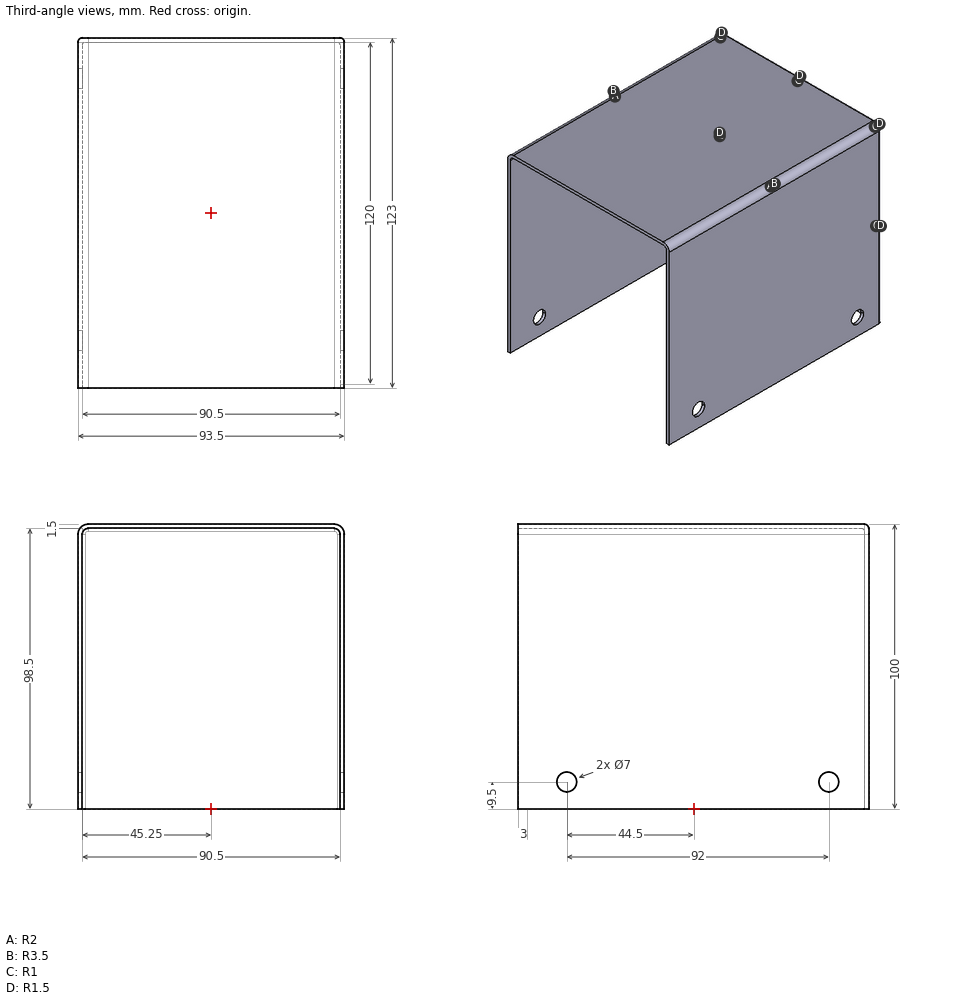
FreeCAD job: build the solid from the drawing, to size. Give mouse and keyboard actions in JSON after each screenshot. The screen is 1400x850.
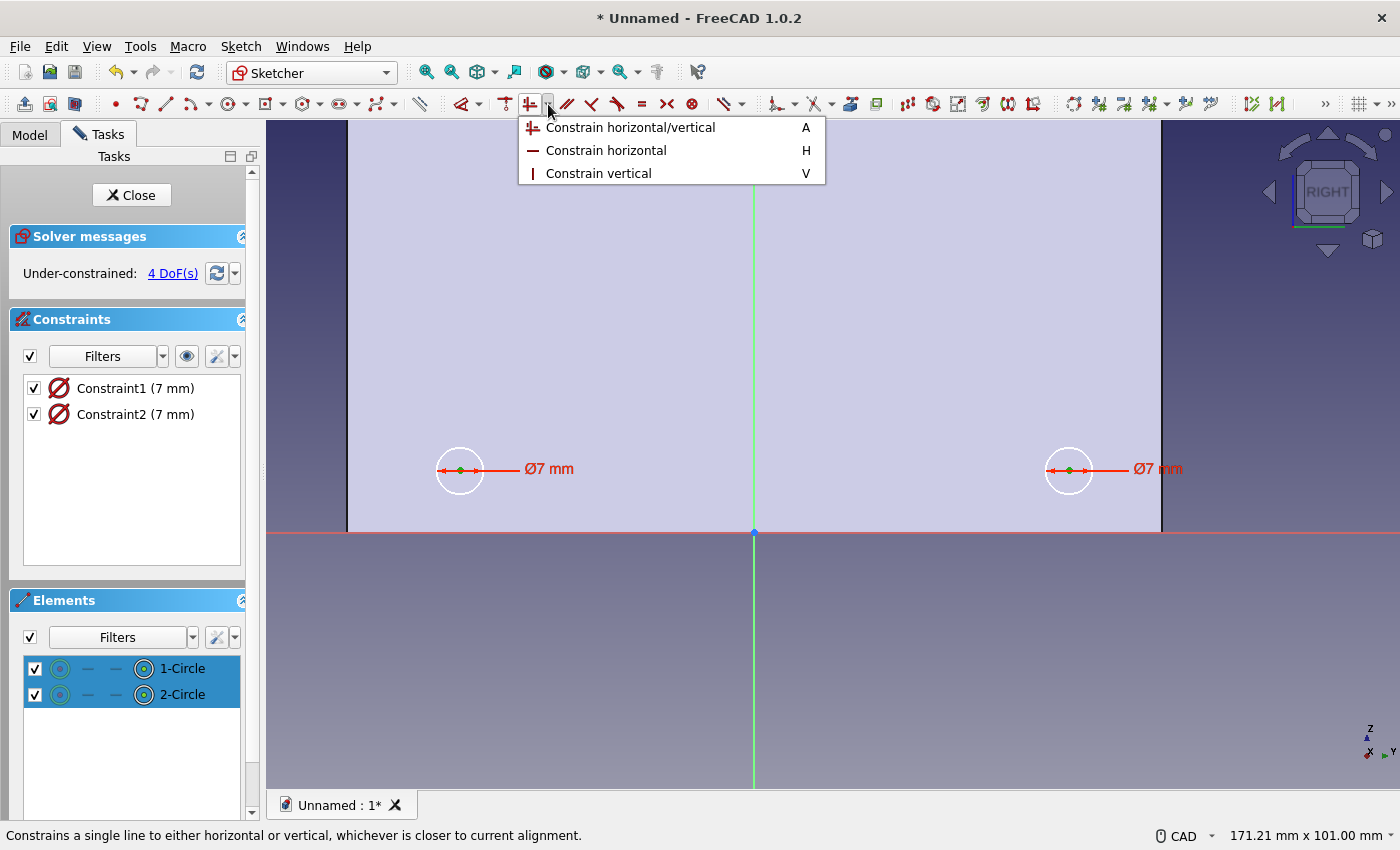
{"action": "left_click", "coordinate": [672, 150]}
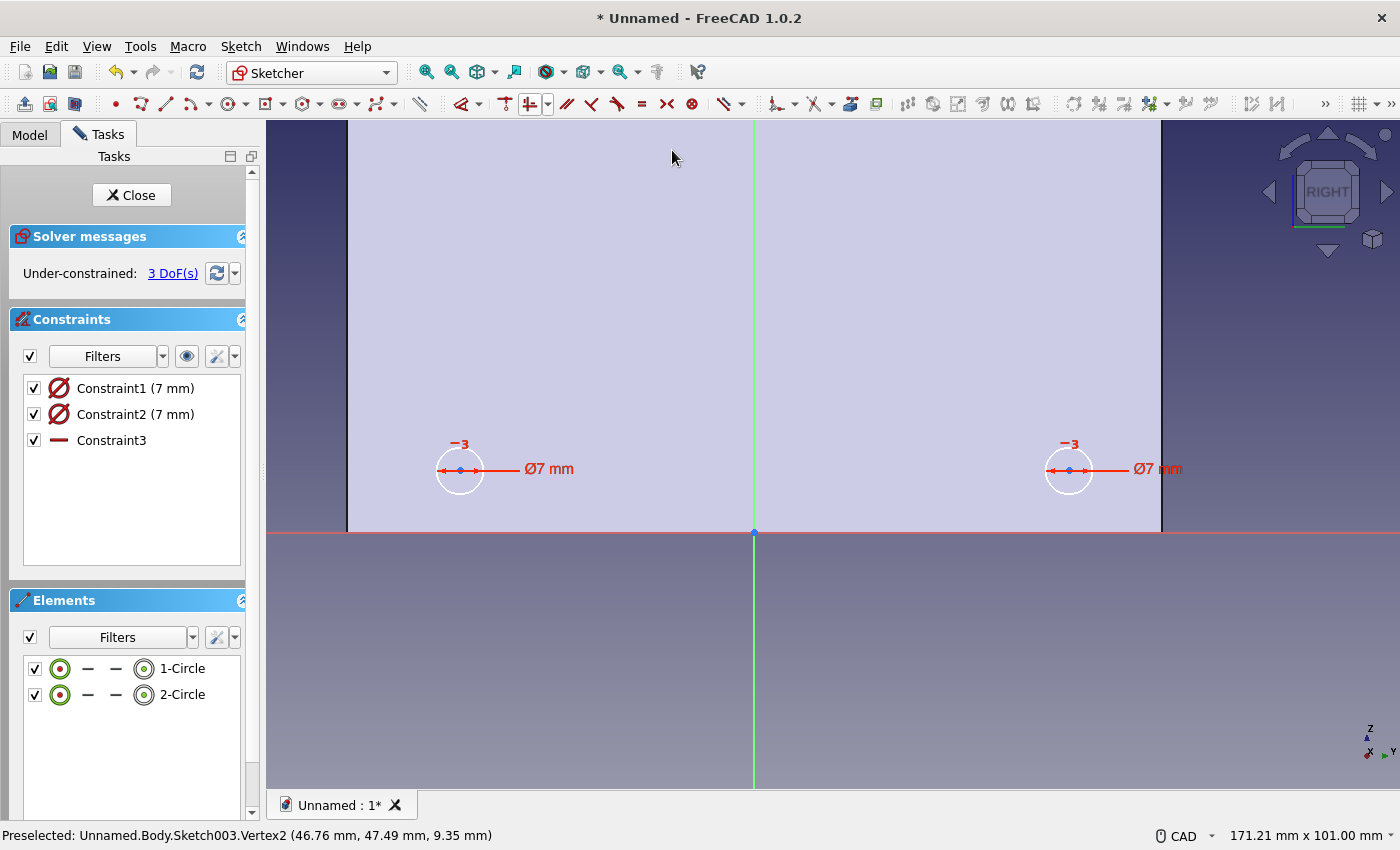
{"action": "left_click", "coordinate": [460, 104]}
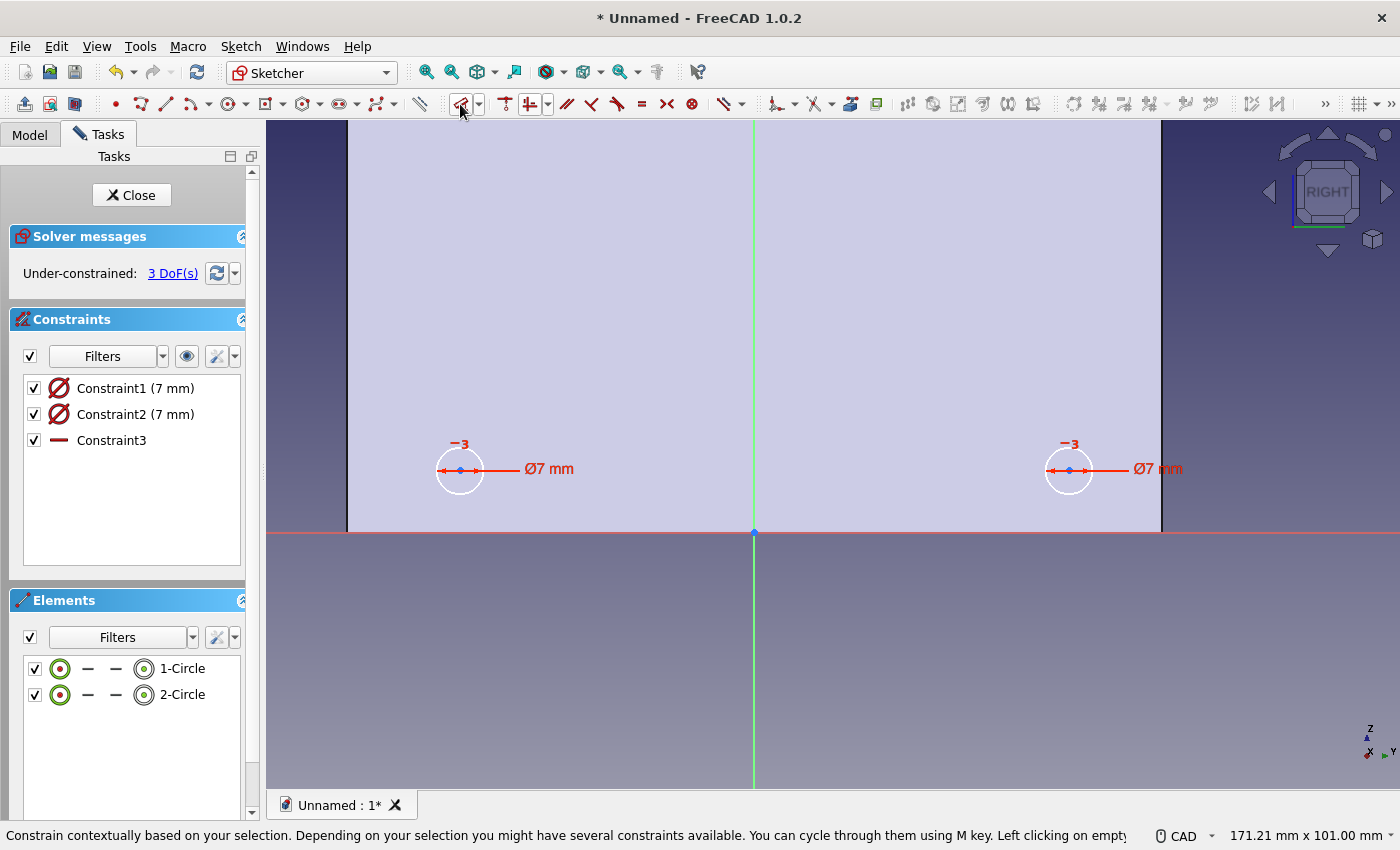
{"action": "left_click", "coordinate": [460, 471]}
{"action": "left_click", "coordinate": [426, 502]}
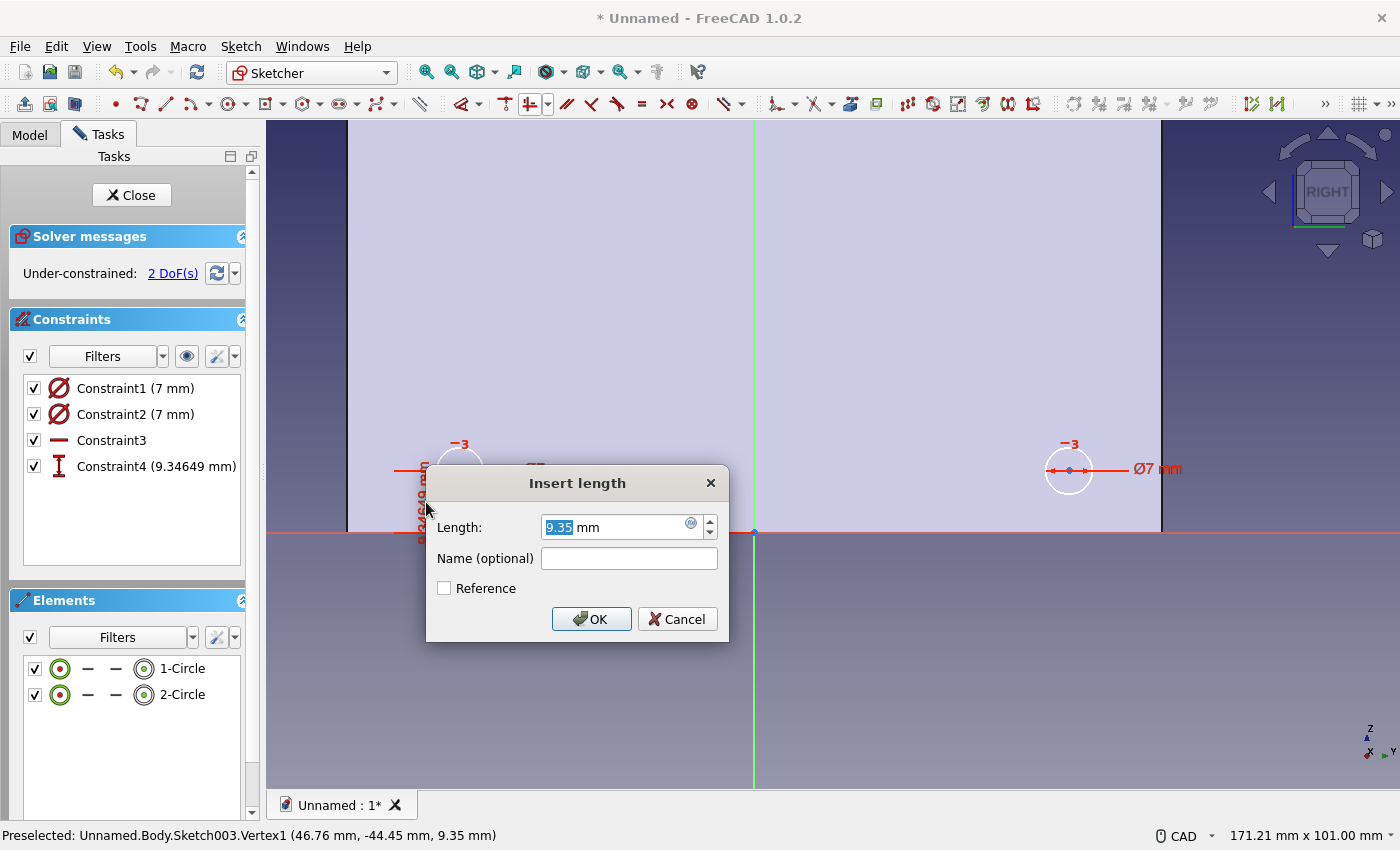
{"action": "type", "text": "9.5"}
{"action": "key", "text": "Return"}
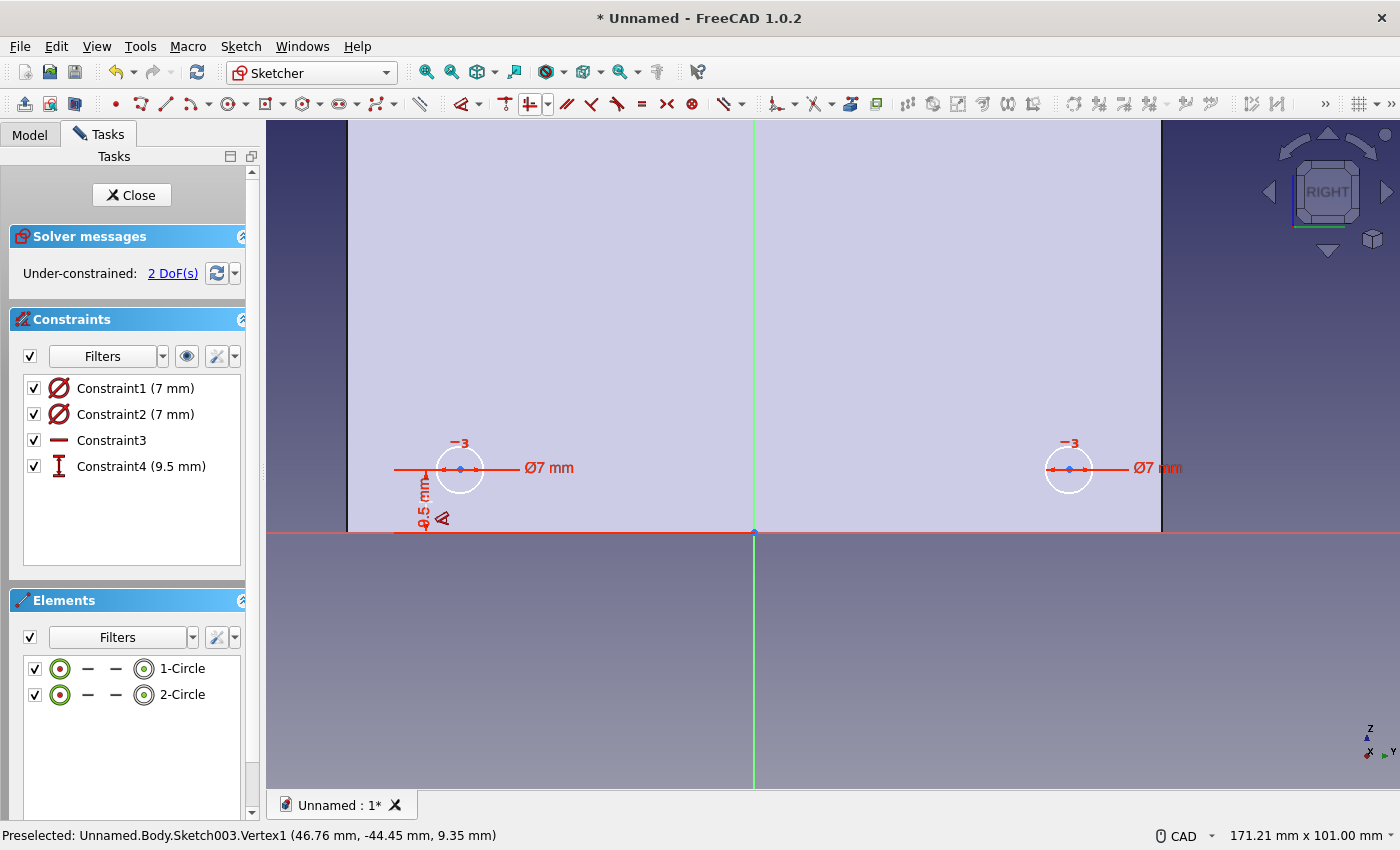
{"action": "left_click", "coordinate": [460, 470]}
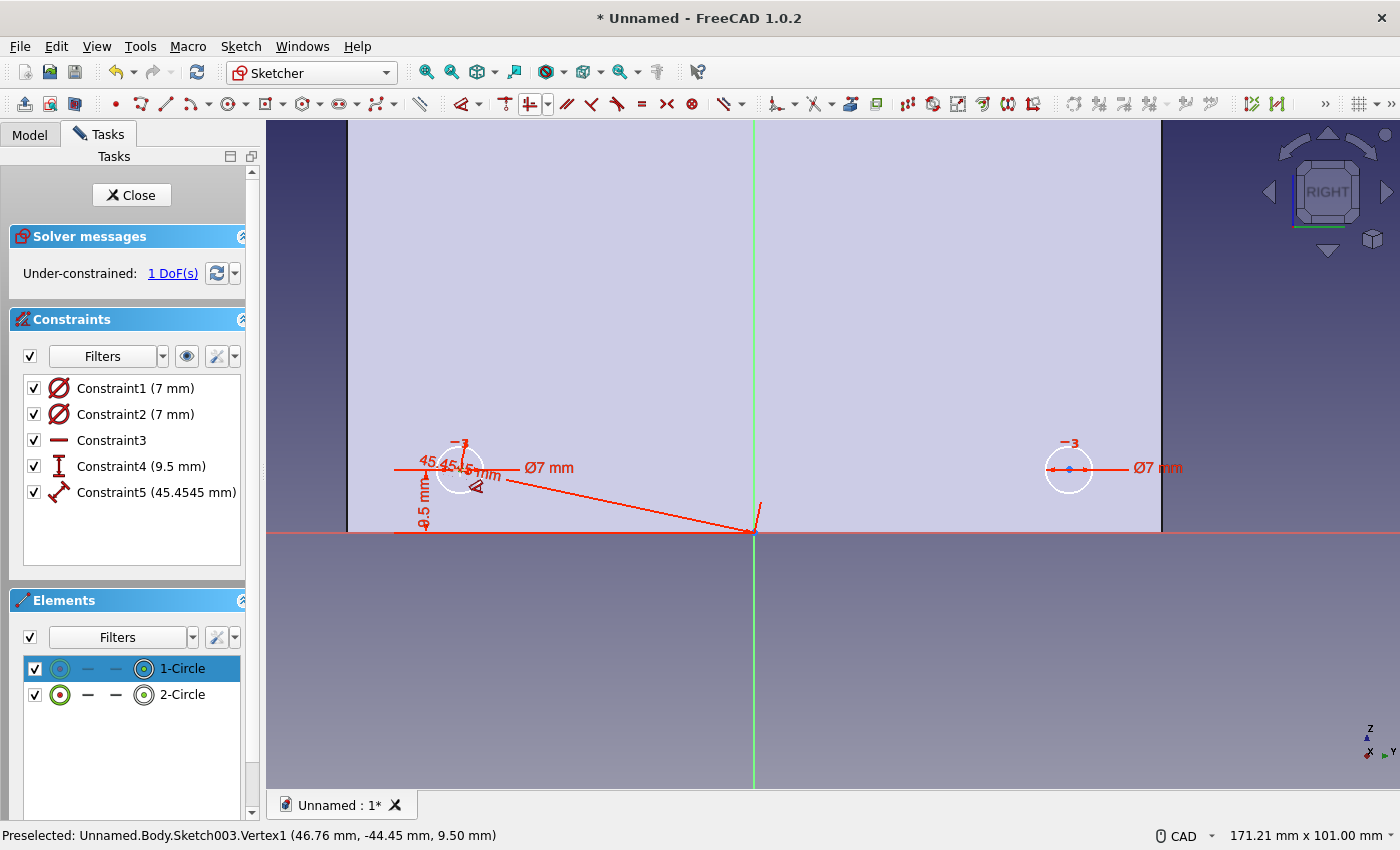
{"action": "left_click", "coordinate": [1069, 470]}
{"action": "left_click", "coordinate": [624, 436]}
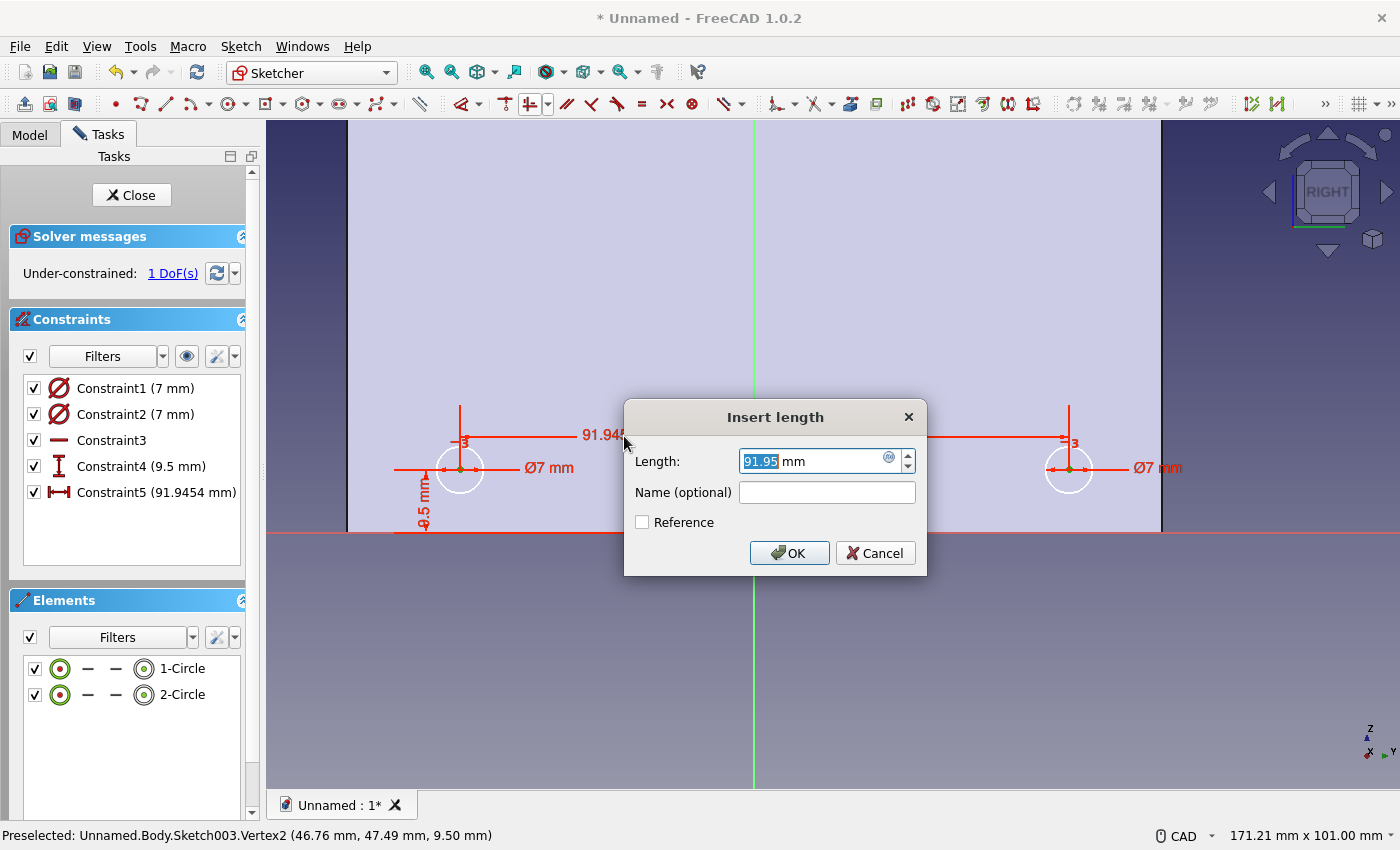
{"action": "type", "text": "92"}
{"action": "key", "text": "Return"}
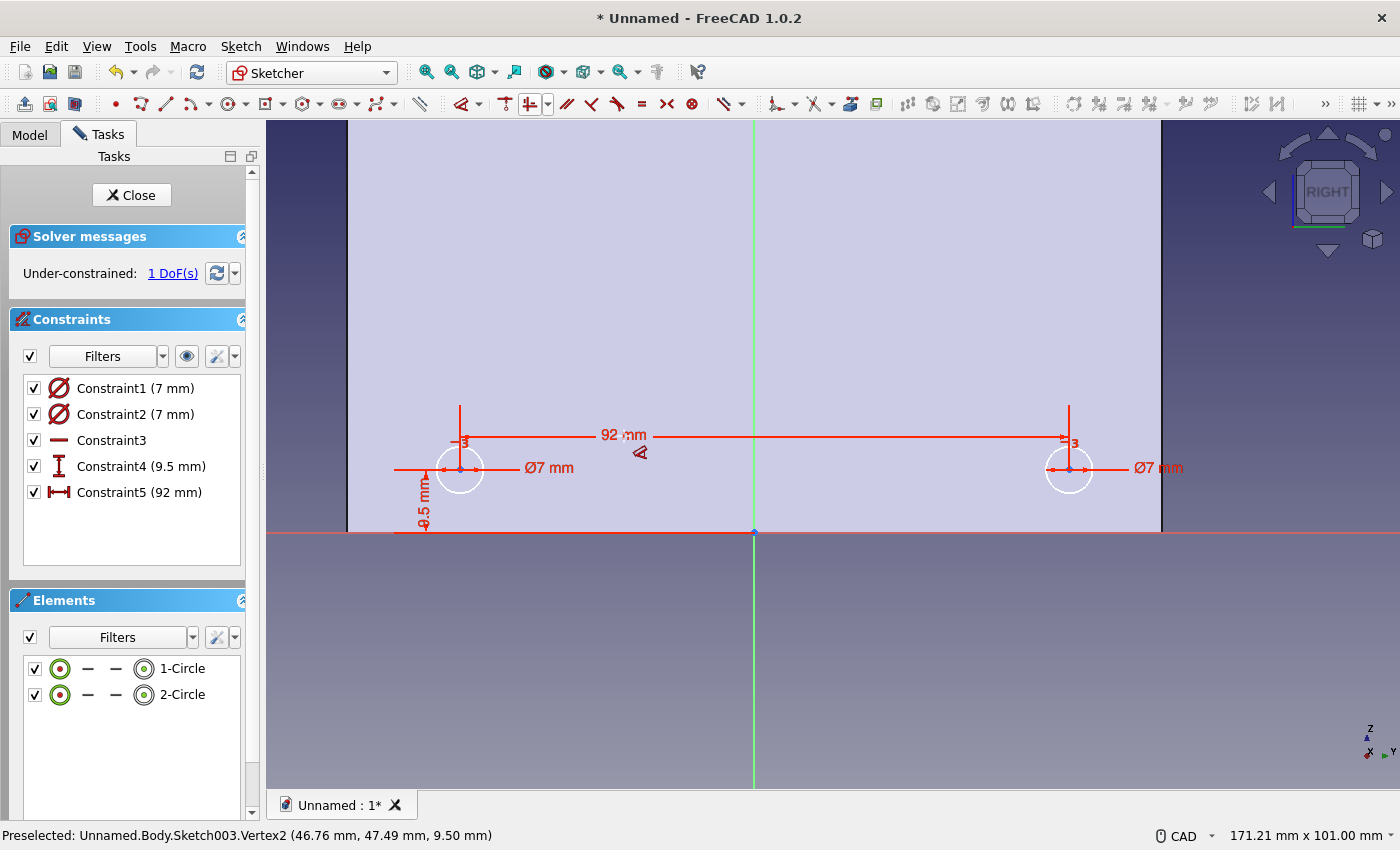
{"action": "left_click", "coordinate": [460, 470]}
{"action": "left_click", "coordinate": [607, 567]}